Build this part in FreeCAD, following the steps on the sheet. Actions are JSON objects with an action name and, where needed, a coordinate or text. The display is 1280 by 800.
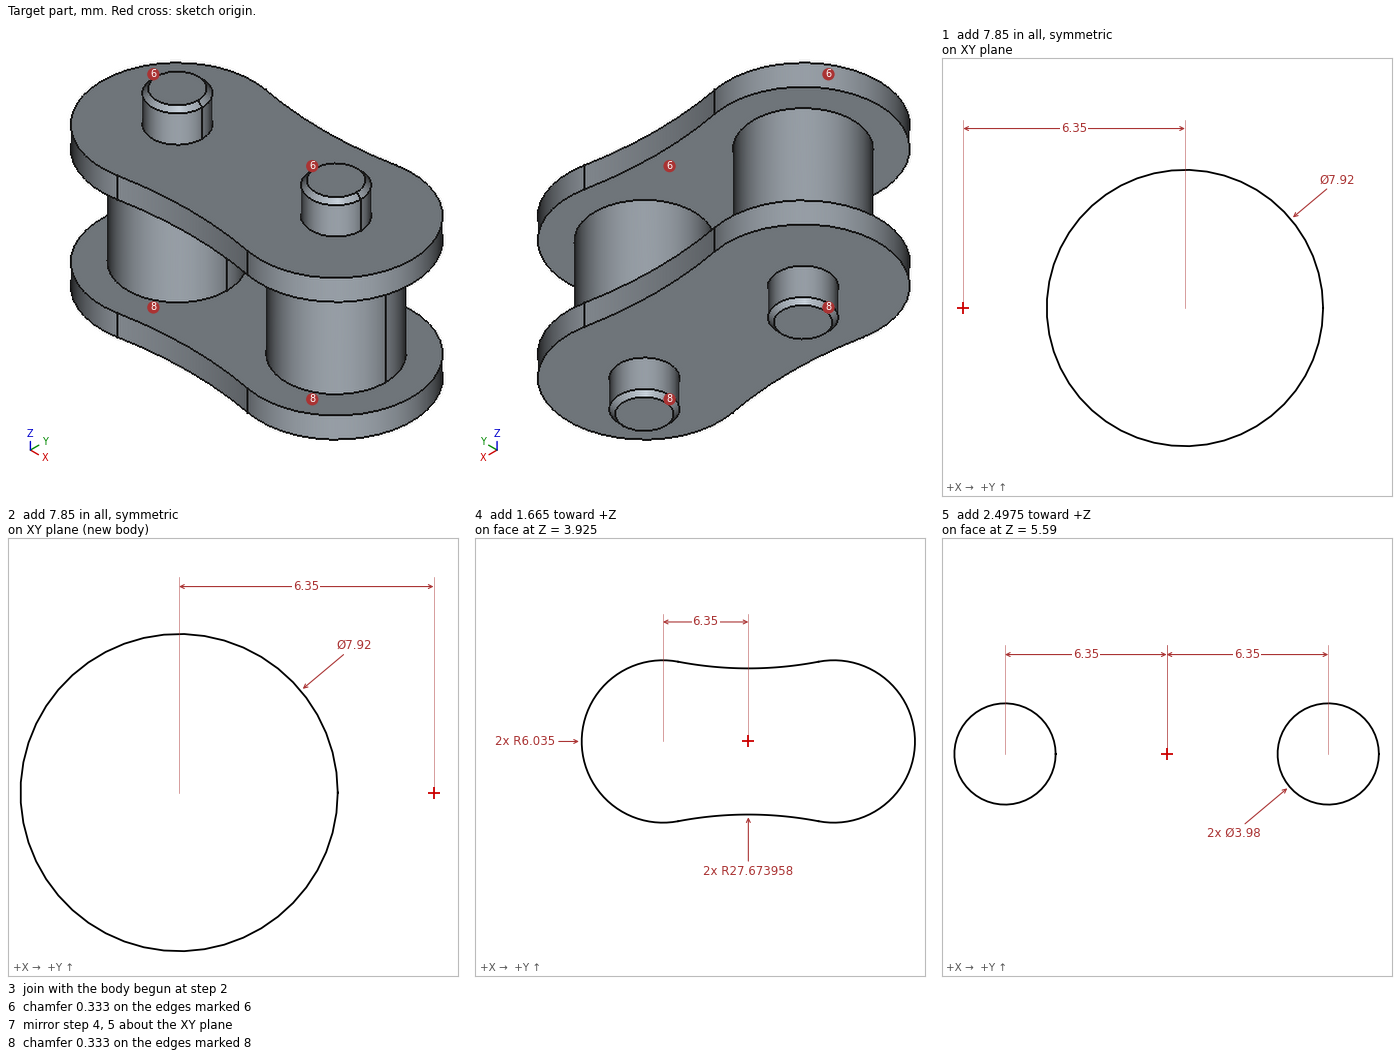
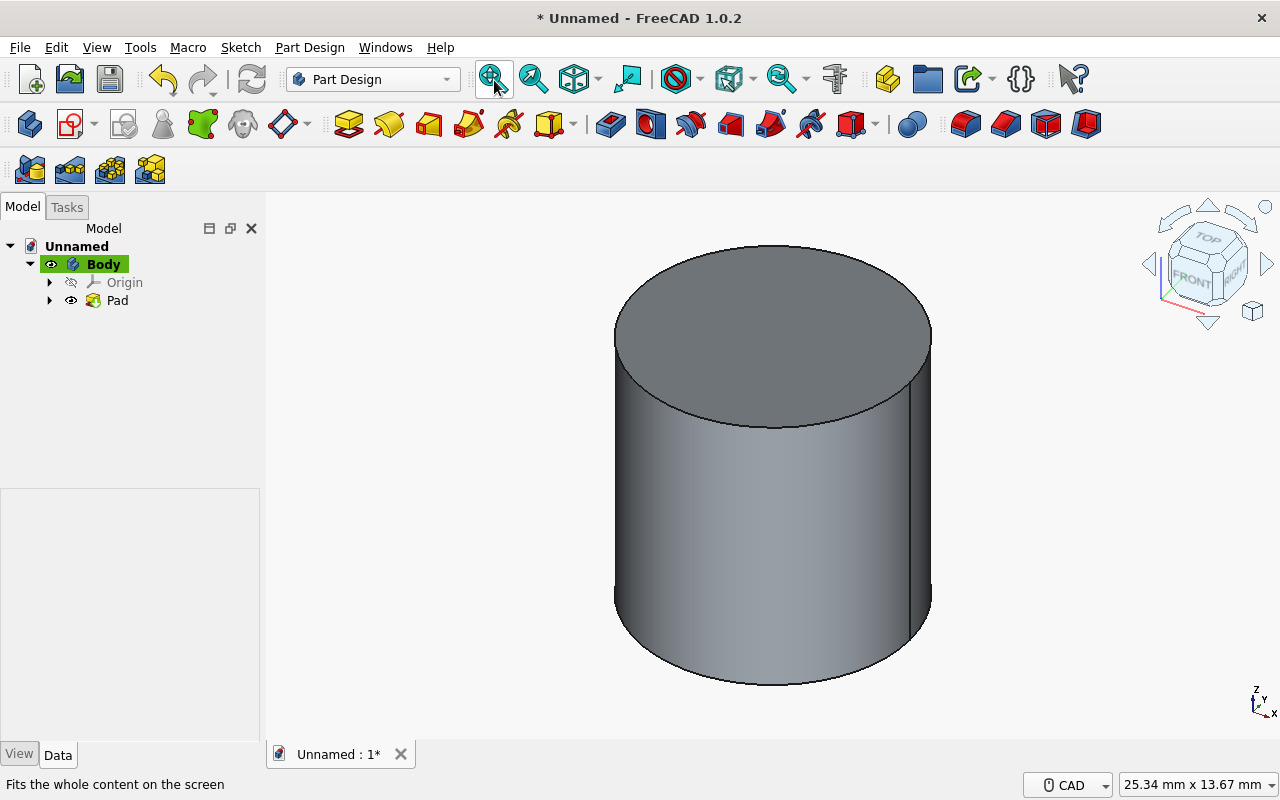
{"action": "left_click", "coordinate": [30, 124]}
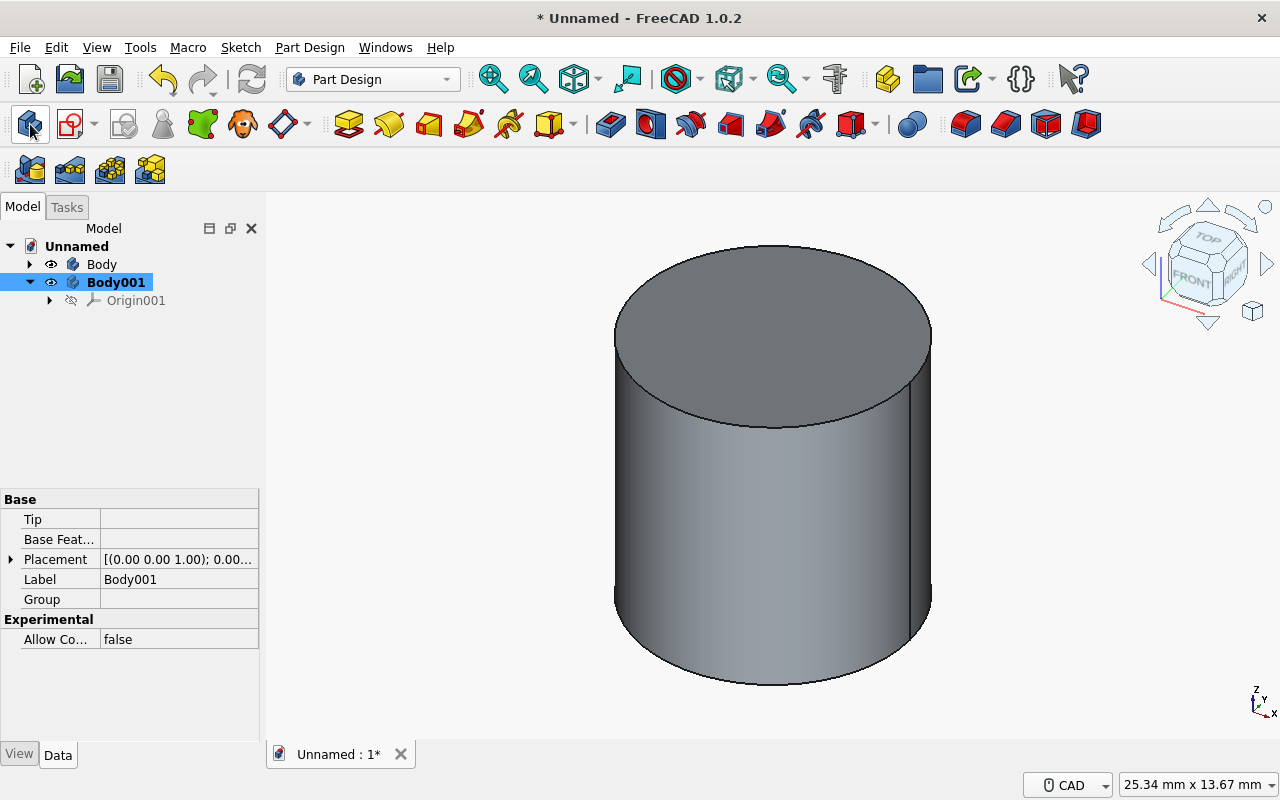
{"action": "left_click", "coordinate": [306, 699]}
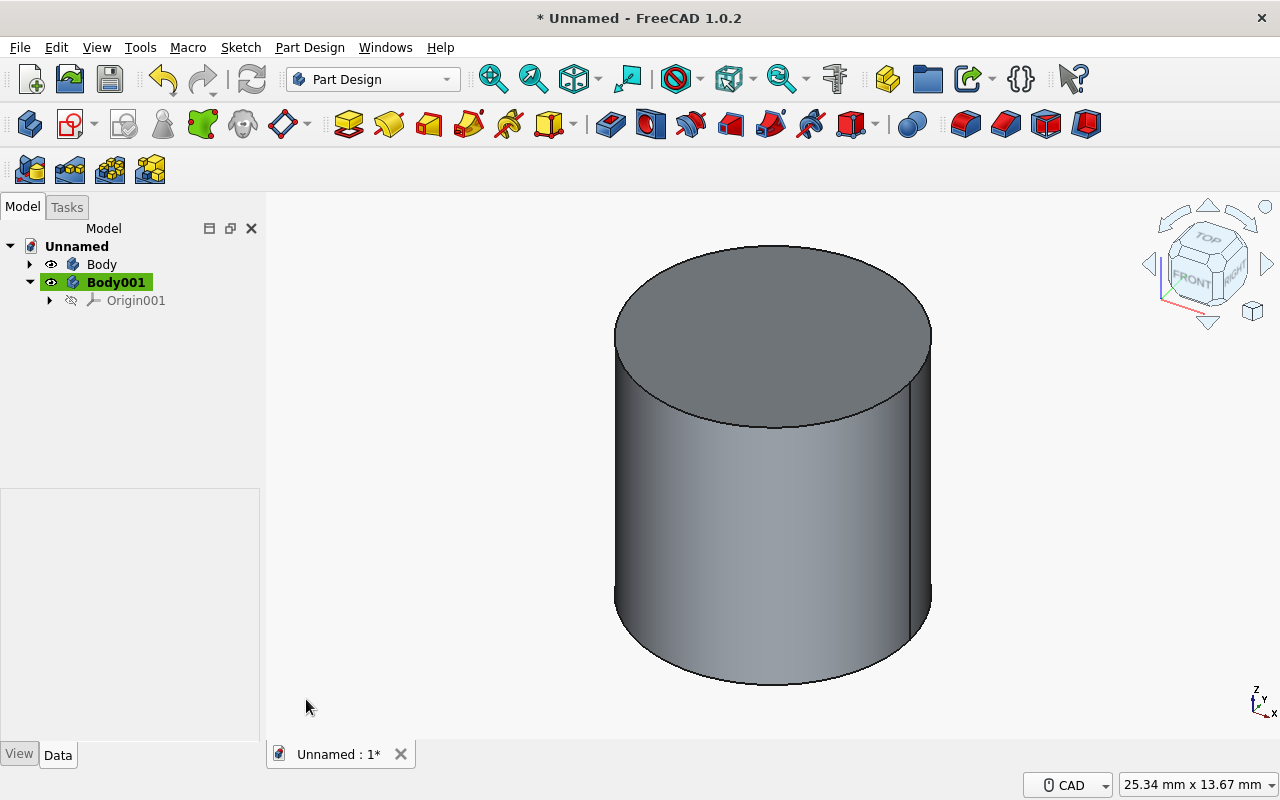
{"action": "left_click", "coordinate": [70, 124]}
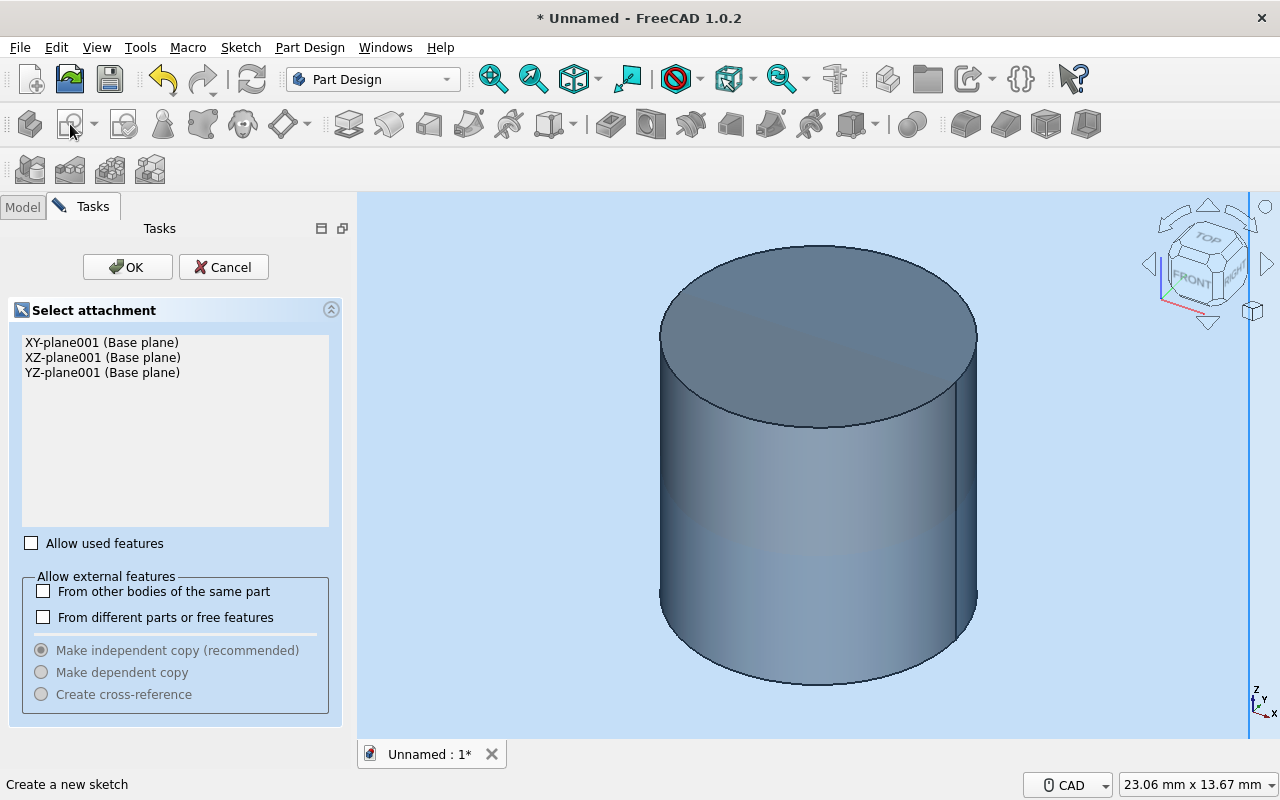
{"action": "left_click", "coordinate": [82, 342]}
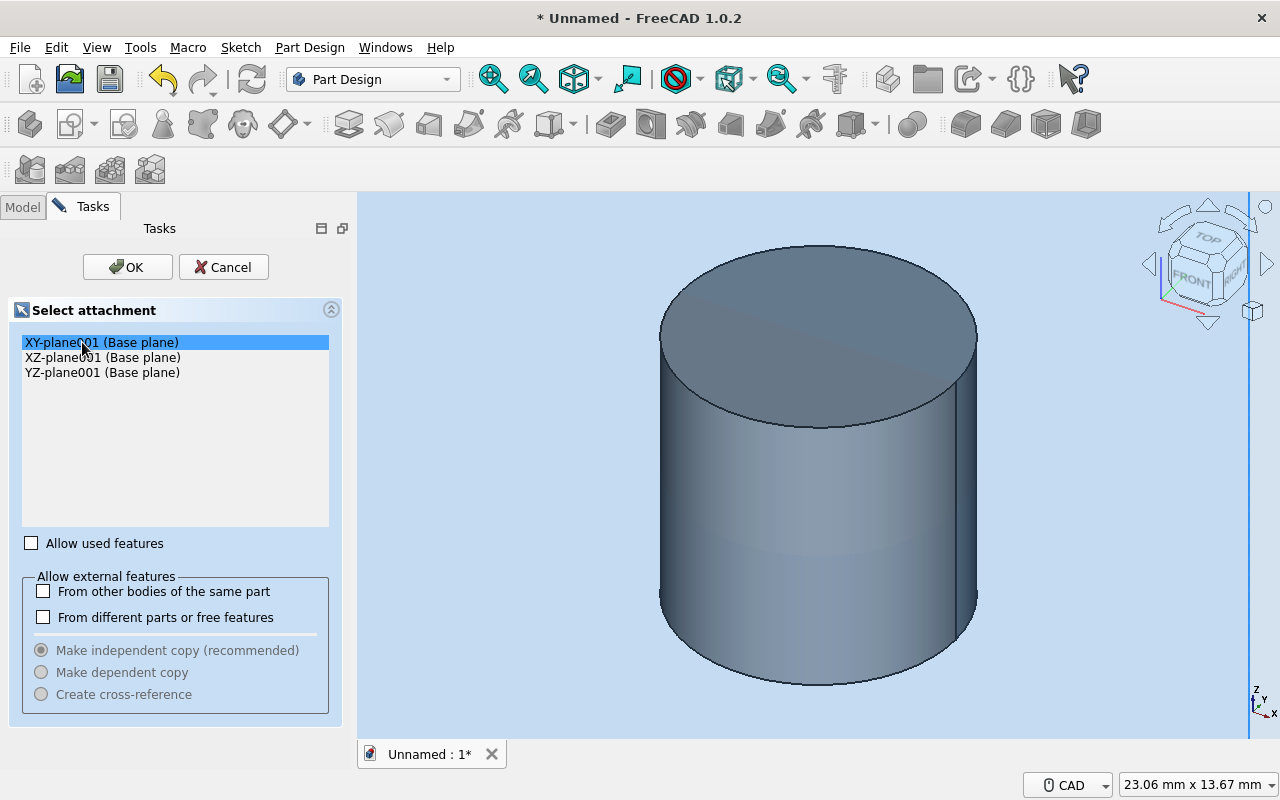
{"action": "left_click", "coordinate": [128, 267]}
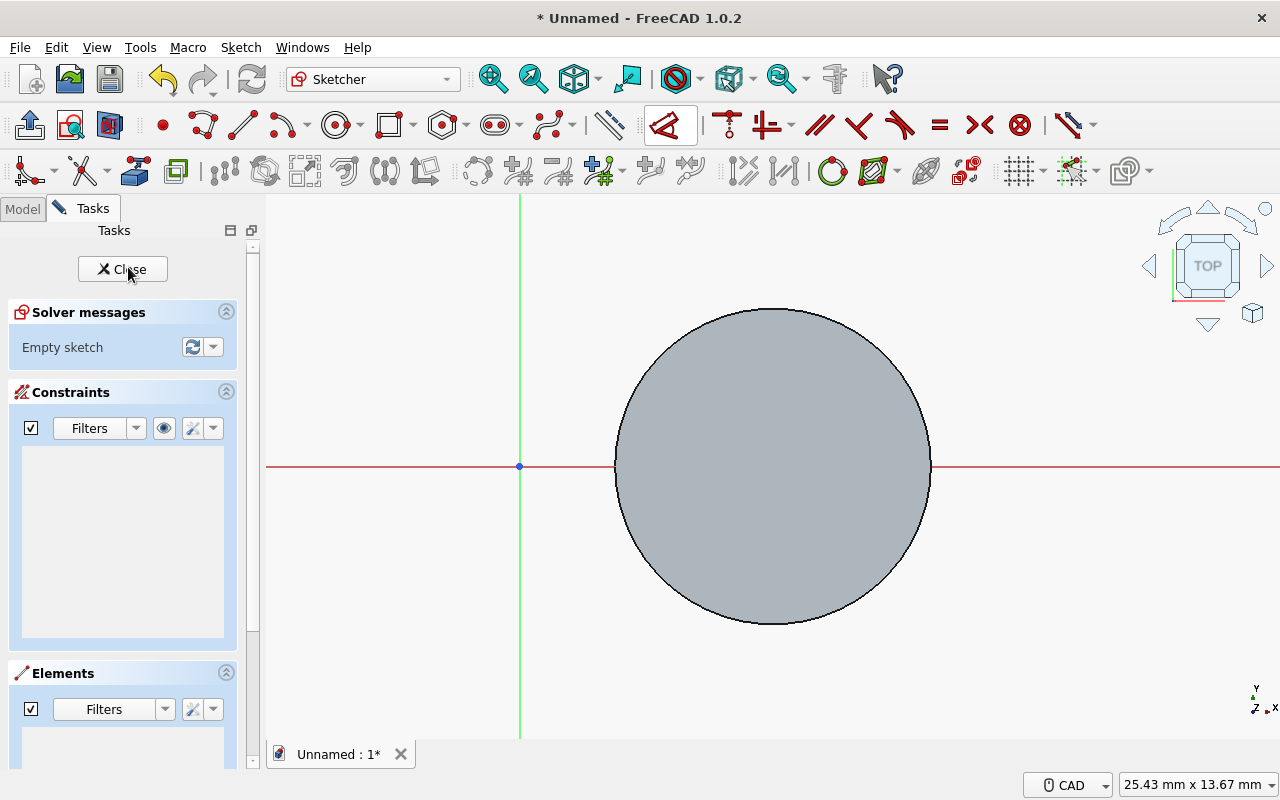
{"action": "scroll", "coordinate": [1115, 466], "scroll_direction": "down", "scroll_amount": 2}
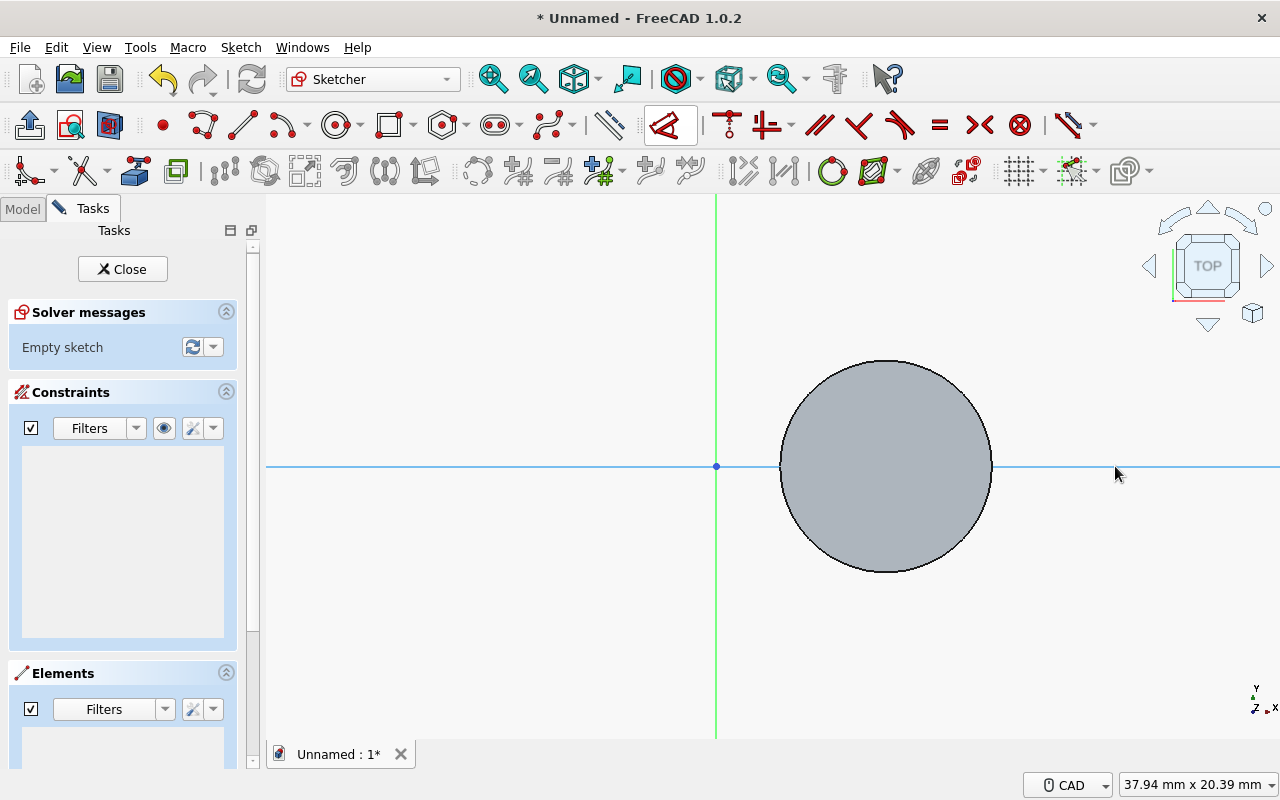
{"action": "scroll", "coordinate": [322, 467], "scroll_direction": "up", "scroll_amount": 2}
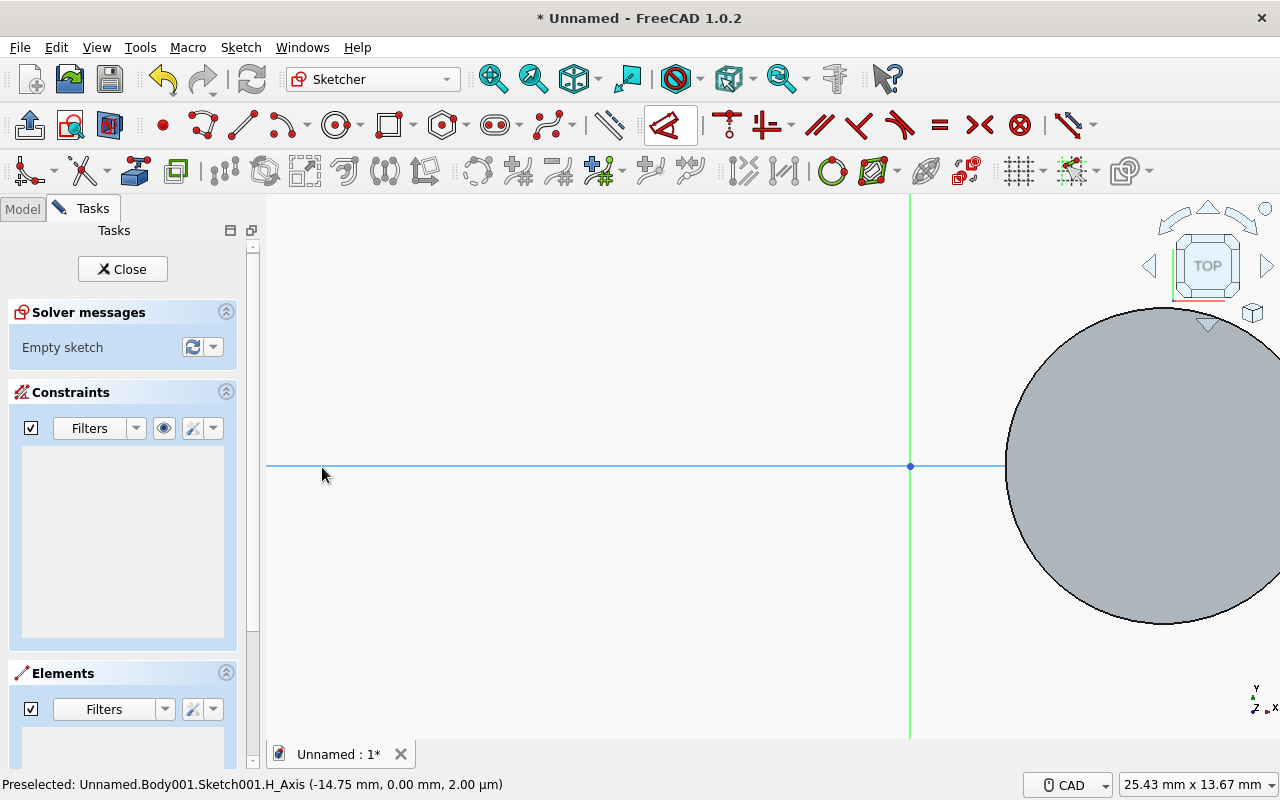
{"action": "left_click", "coordinate": [336, 126]}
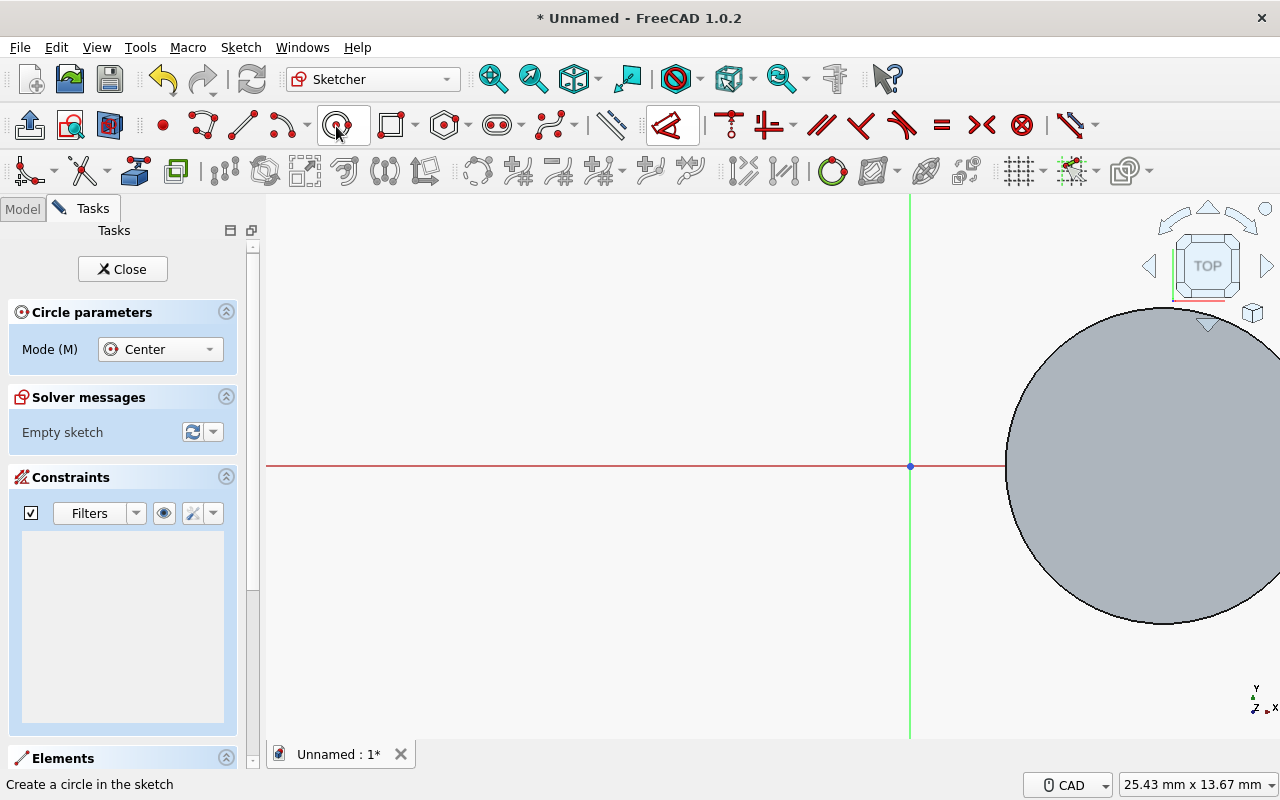
{"action": "left_click", "coordinate": [657, 466]}
{"action": "mouse_move", "coordinate": [769, 354]}